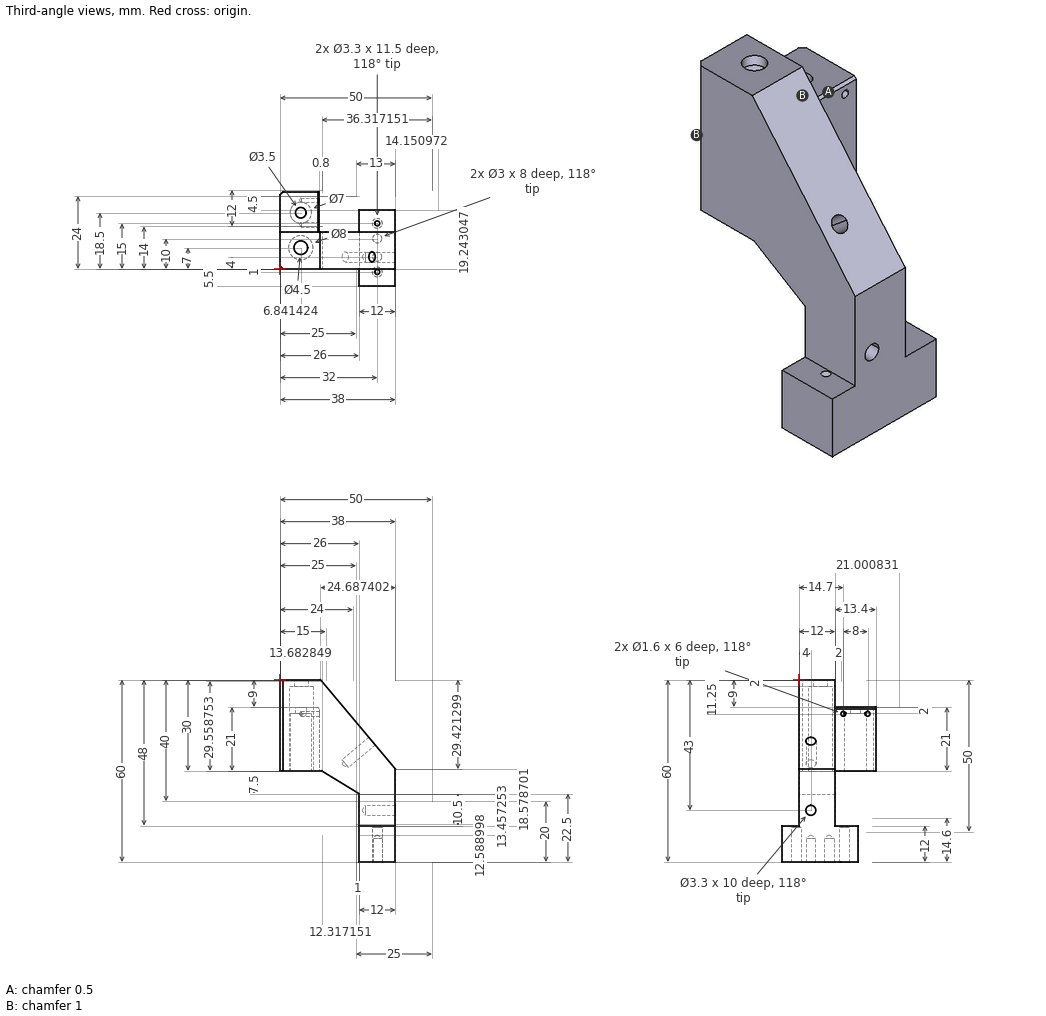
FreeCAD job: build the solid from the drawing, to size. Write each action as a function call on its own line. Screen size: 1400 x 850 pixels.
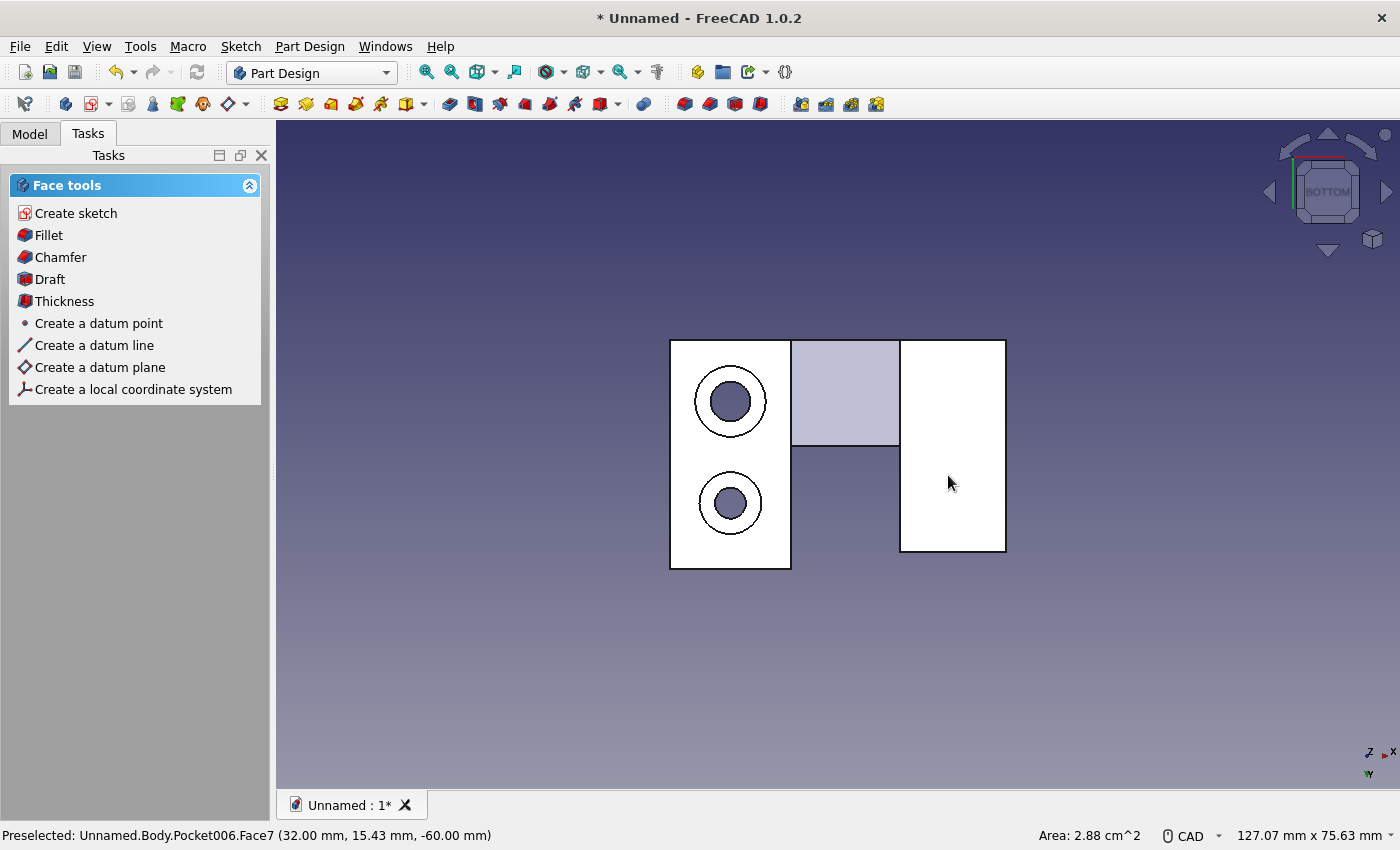
click(90, 104)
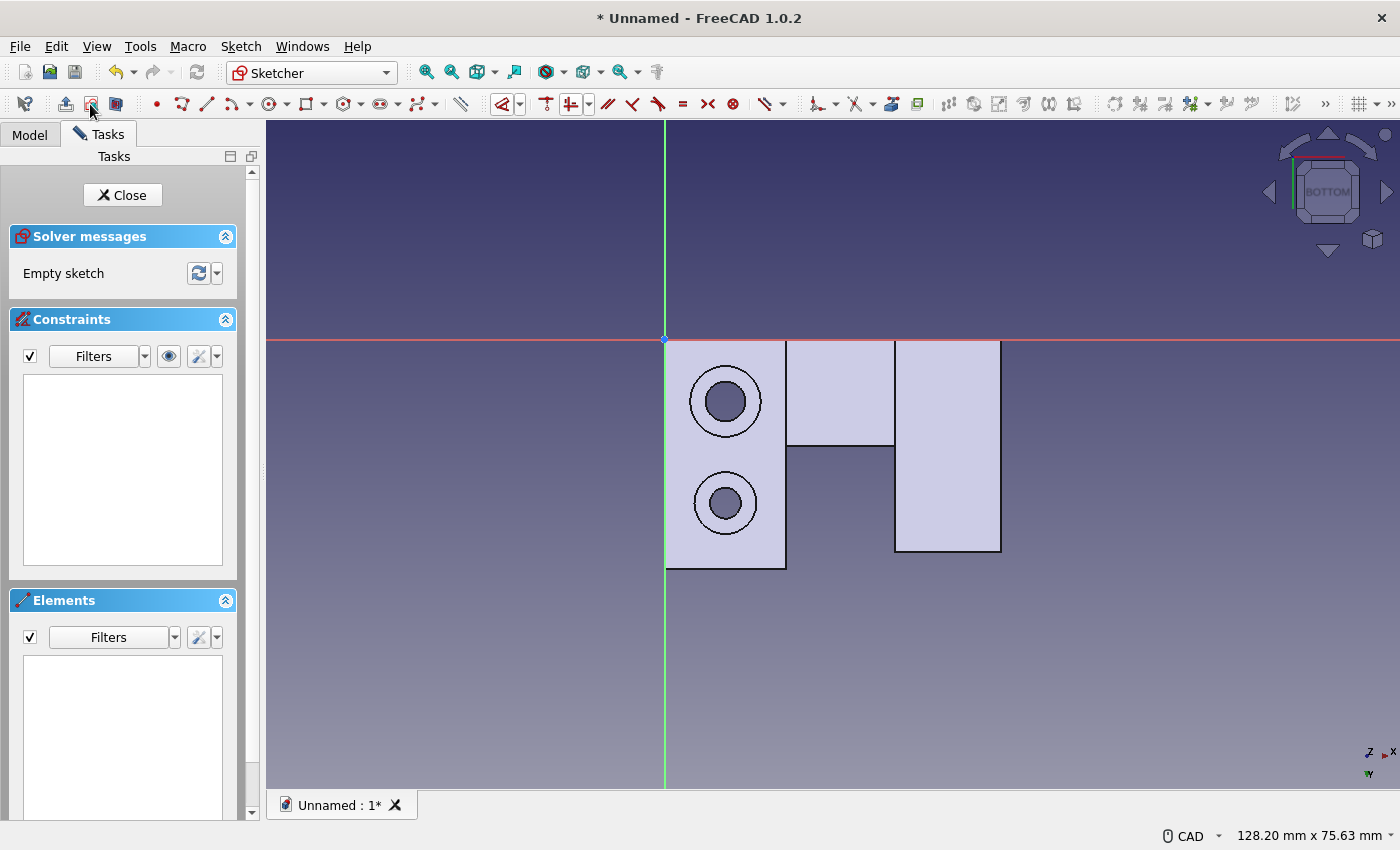
scroll(984, 288, up, 9)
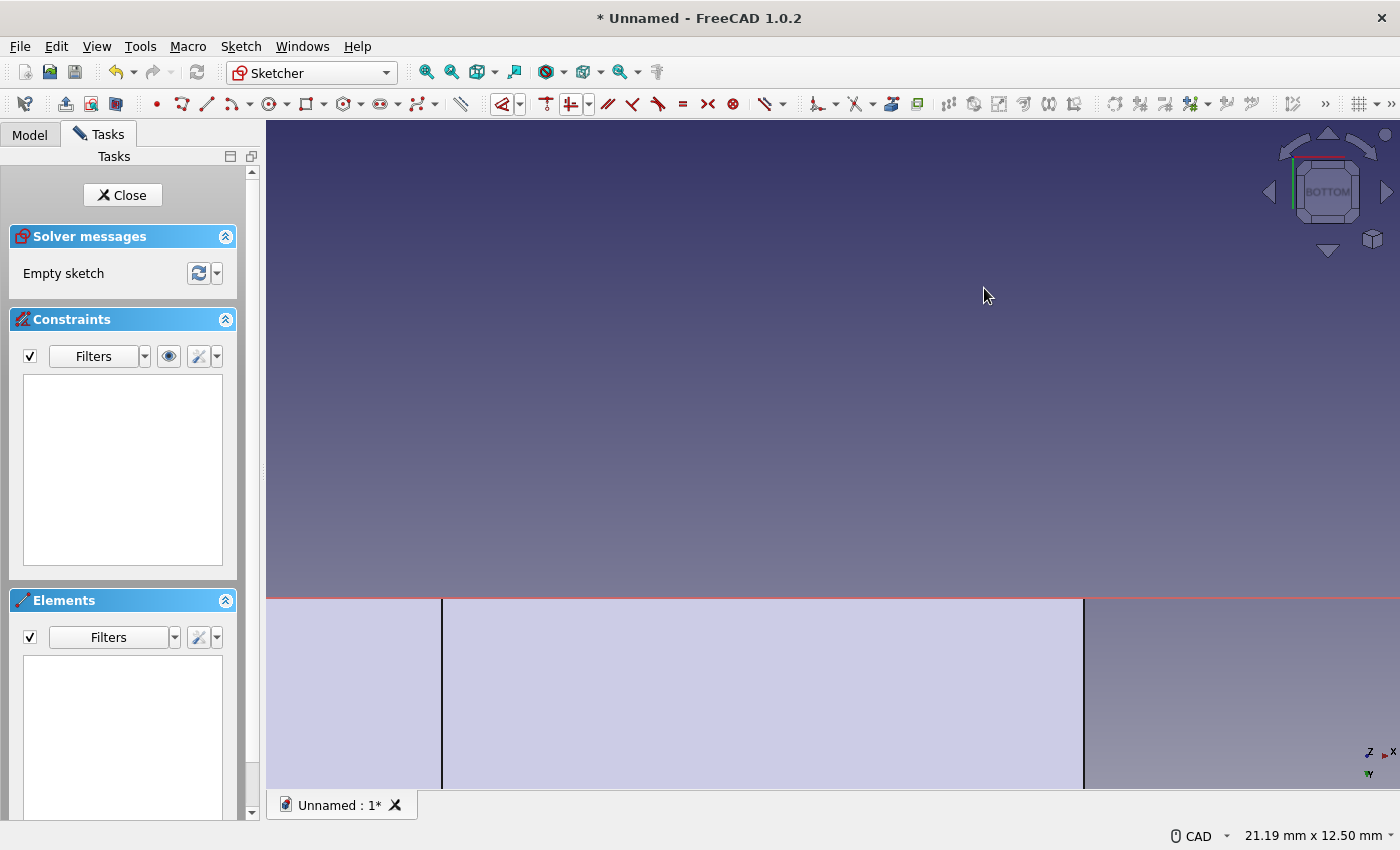
click(306, 104)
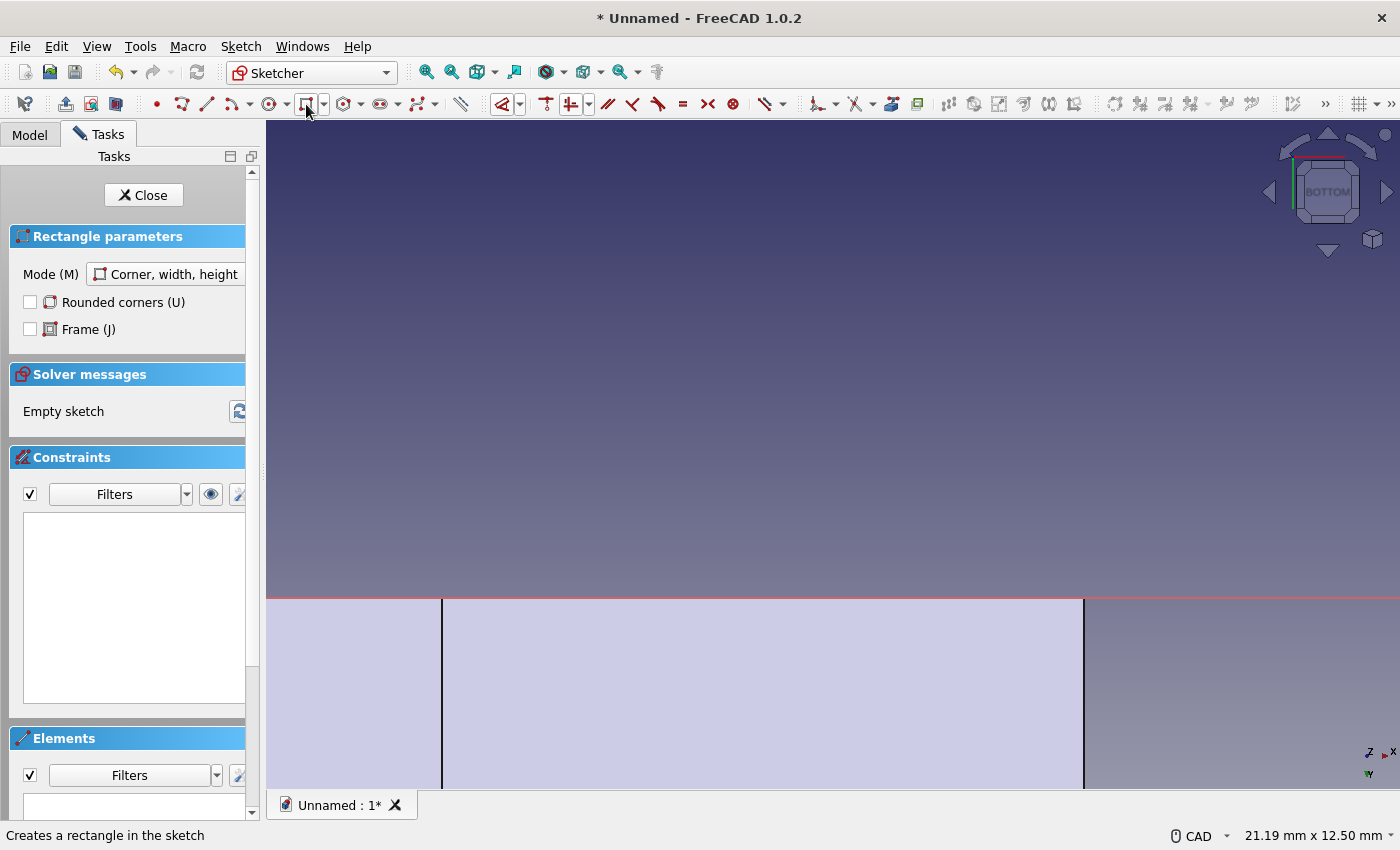
click(442, 304)
click(1084, 598)
key(Escape)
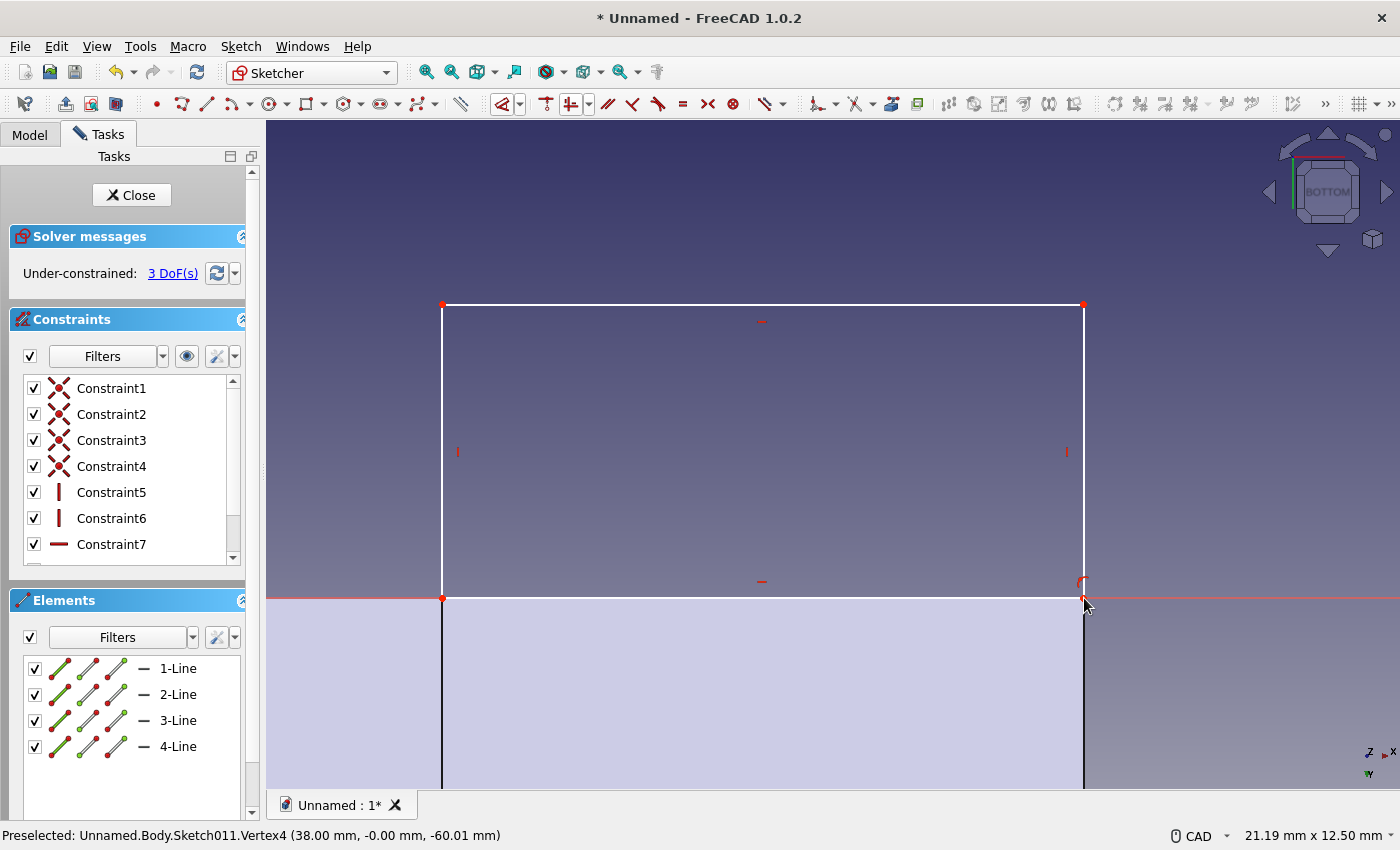
click(635, 598)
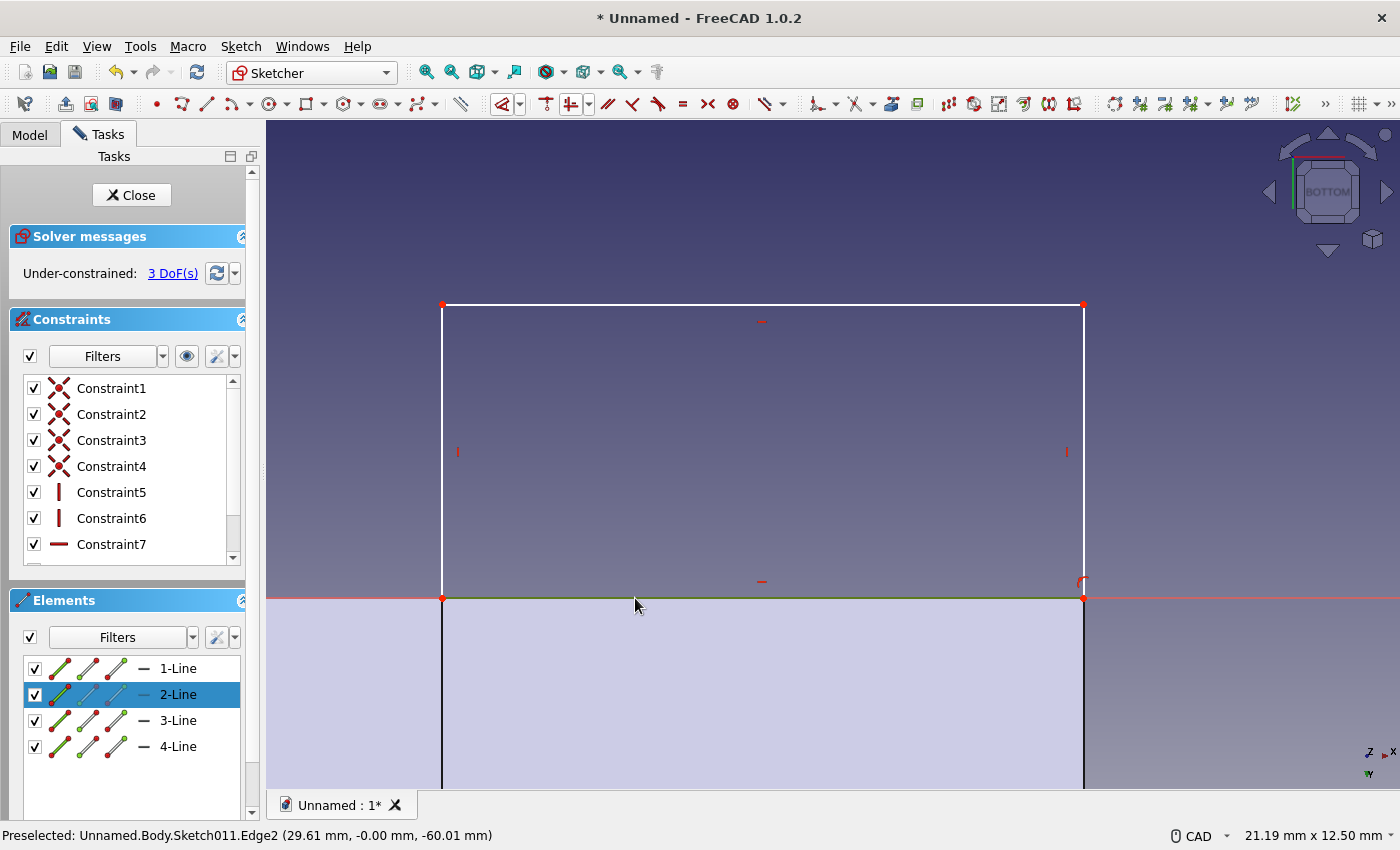
click(520, 104)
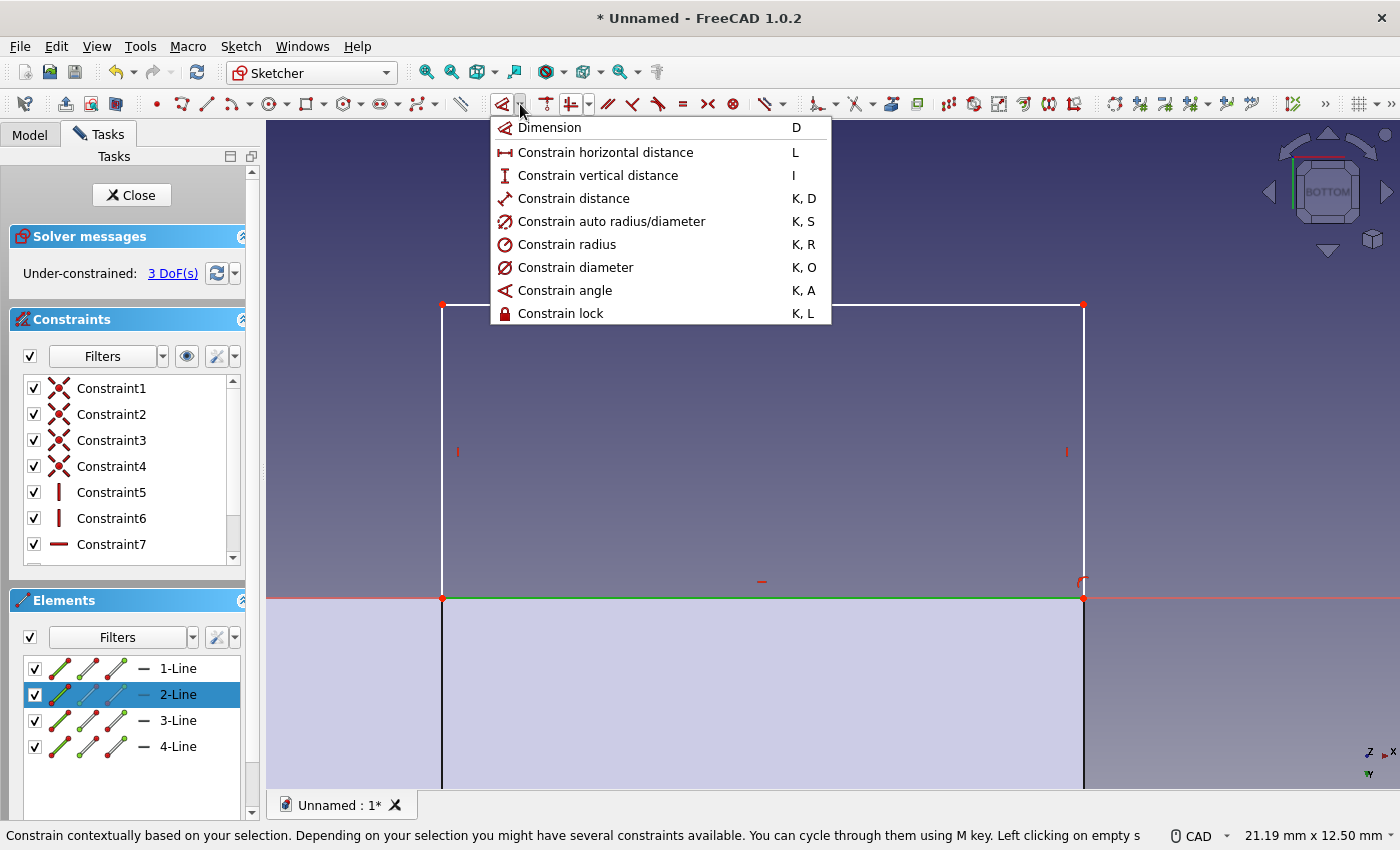
click(661, 152)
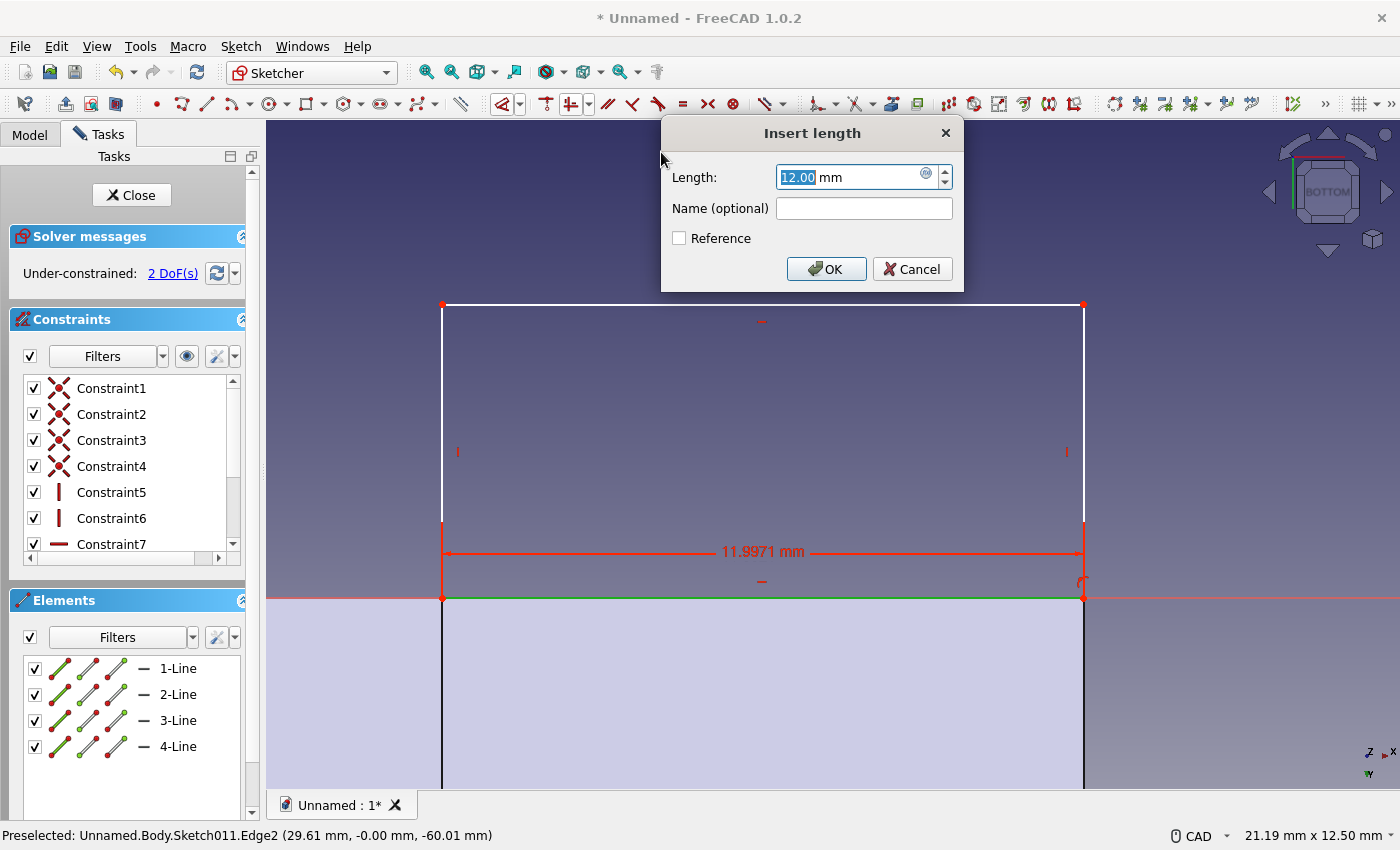
text(12)
key(Return)